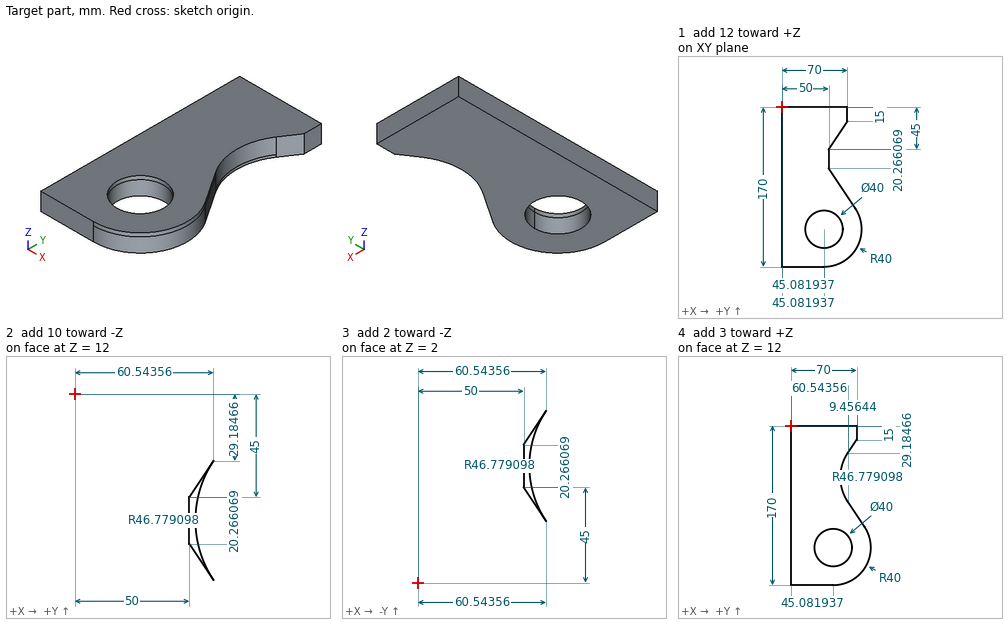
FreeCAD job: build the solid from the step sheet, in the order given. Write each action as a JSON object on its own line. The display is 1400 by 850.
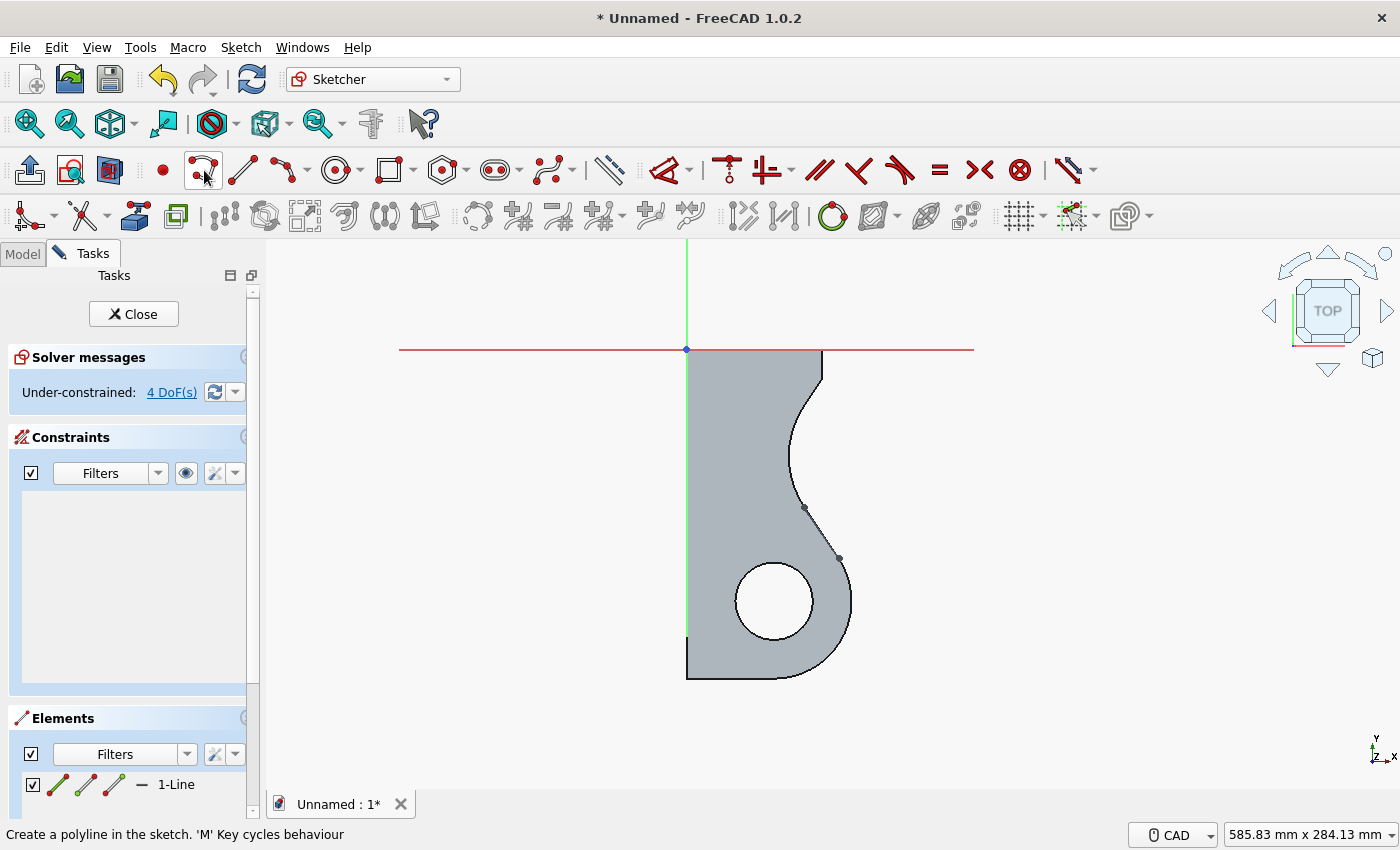
{"action": "left_click", "coordinate": [804, 406]}
{"action": "left_click", "coordinate": [822, 379]}
{"action": "left_click", "coordinate": [822, 350]}
{"action": "left_click", "coordinate": [687, 350]}
{"action": "left_click", "coordinate": [696, 679]}
{"action": "left_click", "coordinate": [774, 679]}
{"action": "right_click", "coordinate": [774, 679]}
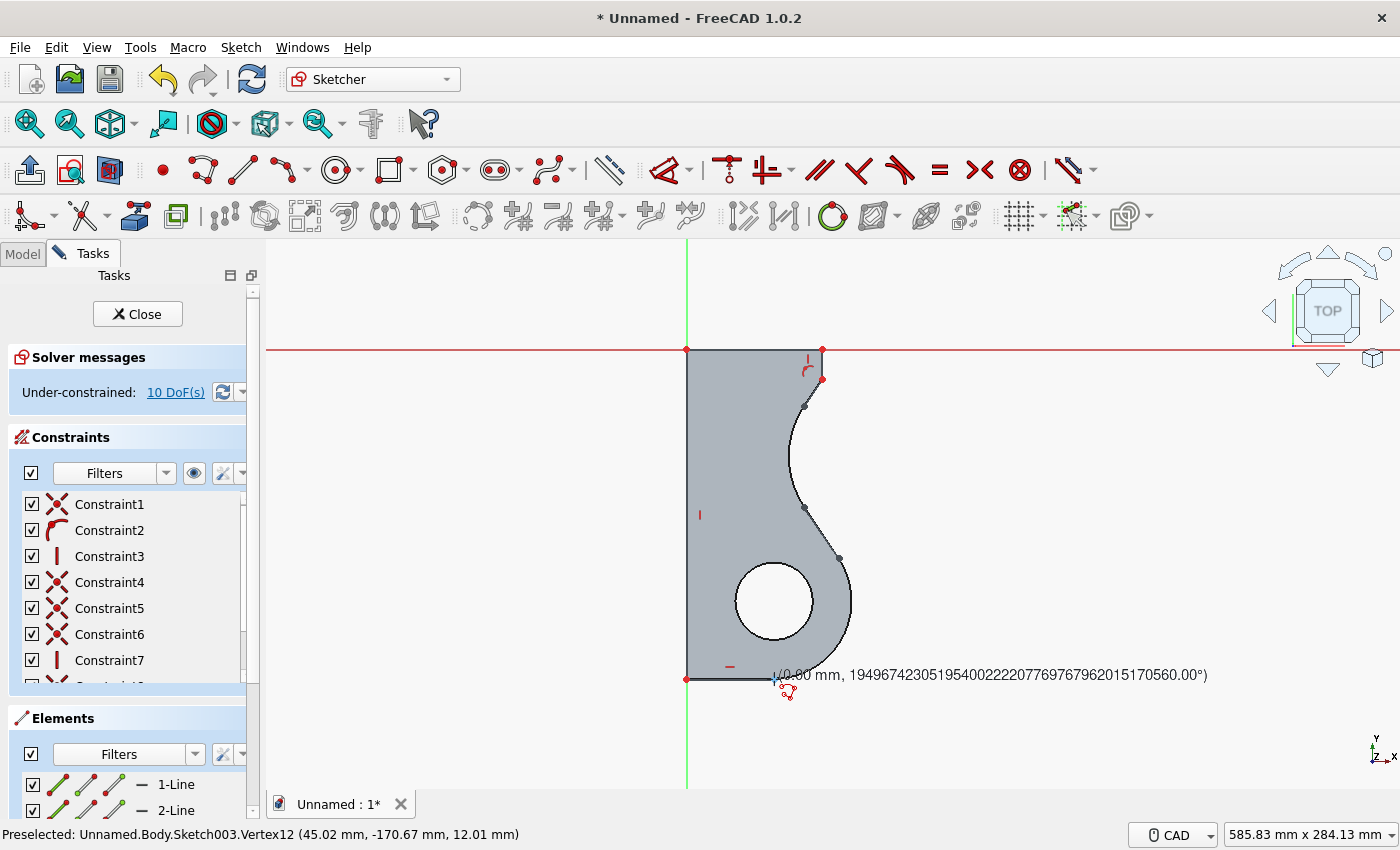
{"action": "left_click", "coordinate": [284, 170]}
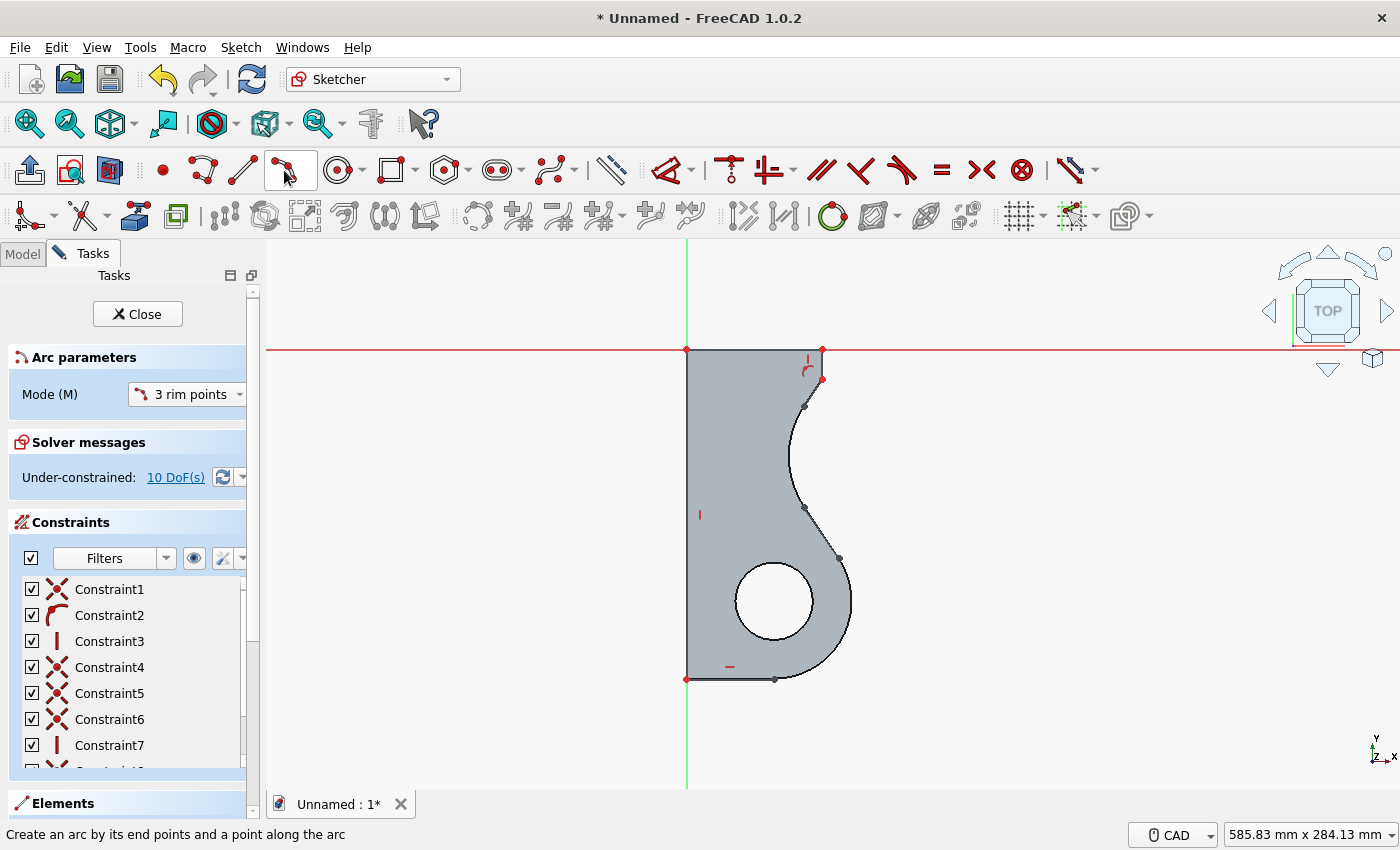
{"action": "left_click", "coordinate": [804, 508]}
{"action": "left_click", "coordinate": [804, 407]}
{"action": "left_click", "coordinate": [789, 456]}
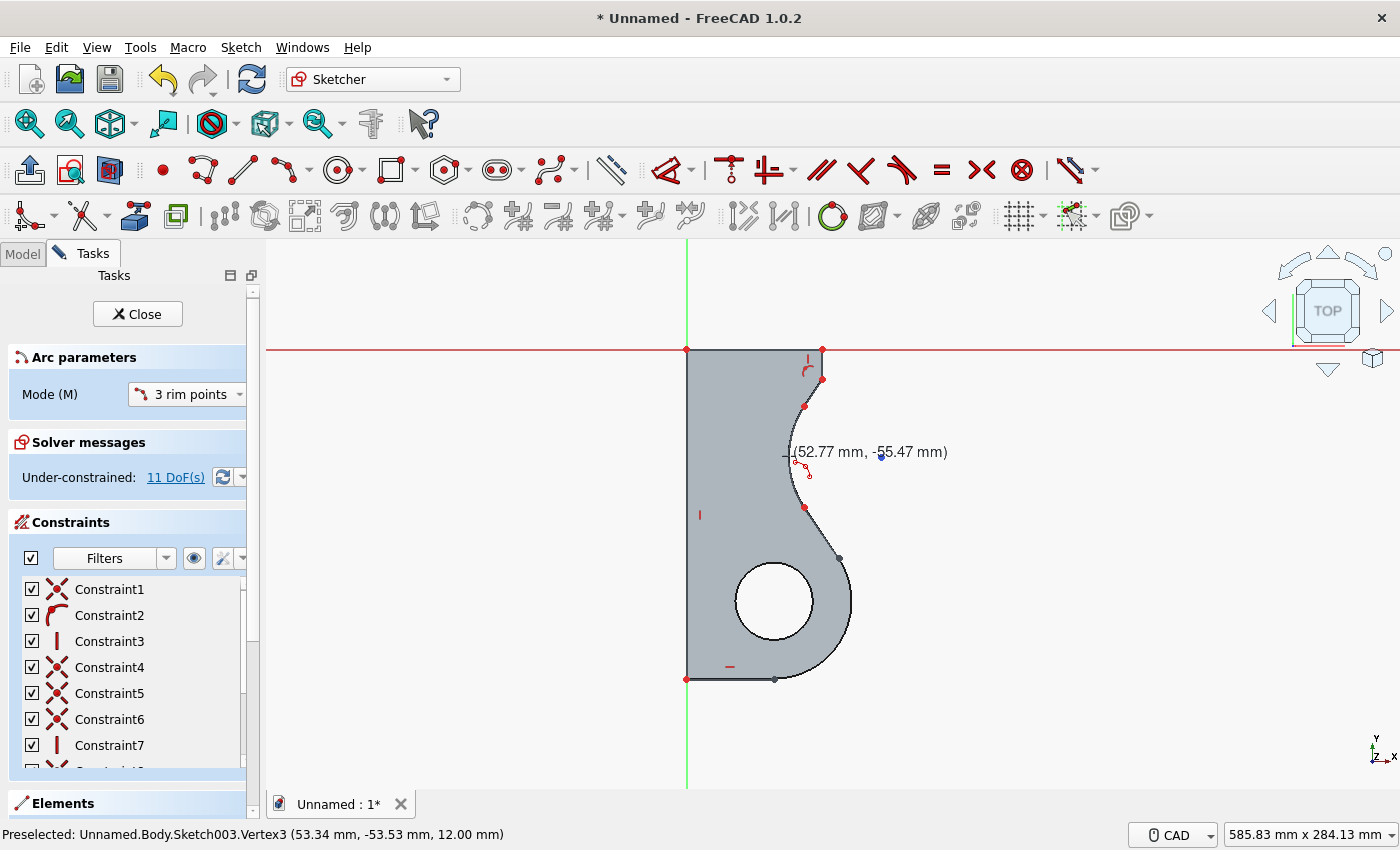
{"action": "left_click", "coordinate": [774, 680]}
{"action": "left_click", "coordinate": [839, 559]}
{"action": "left_click", "coordinate": [842, 638]}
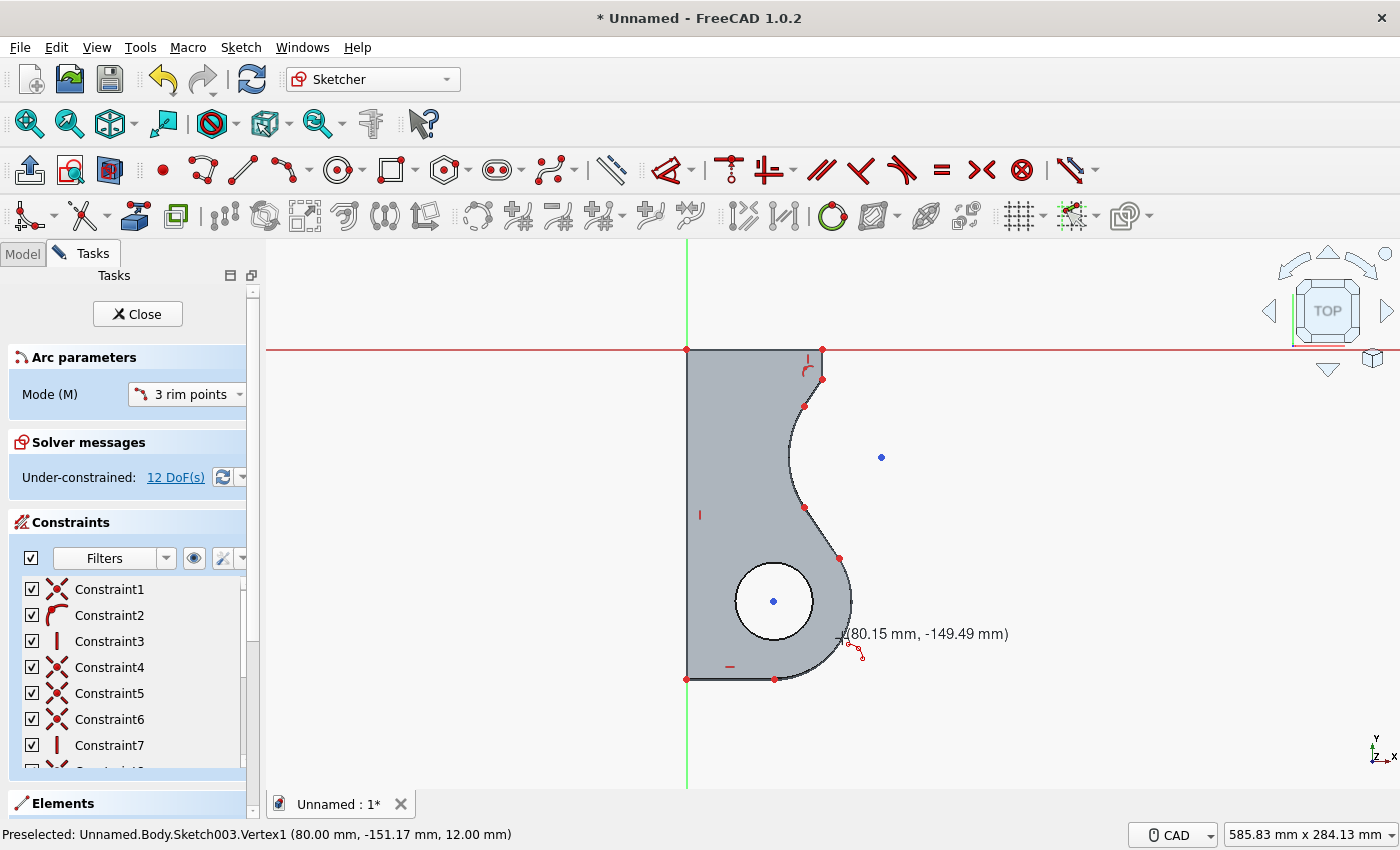
{"action": "left_click", "coordinate": [338, 170]}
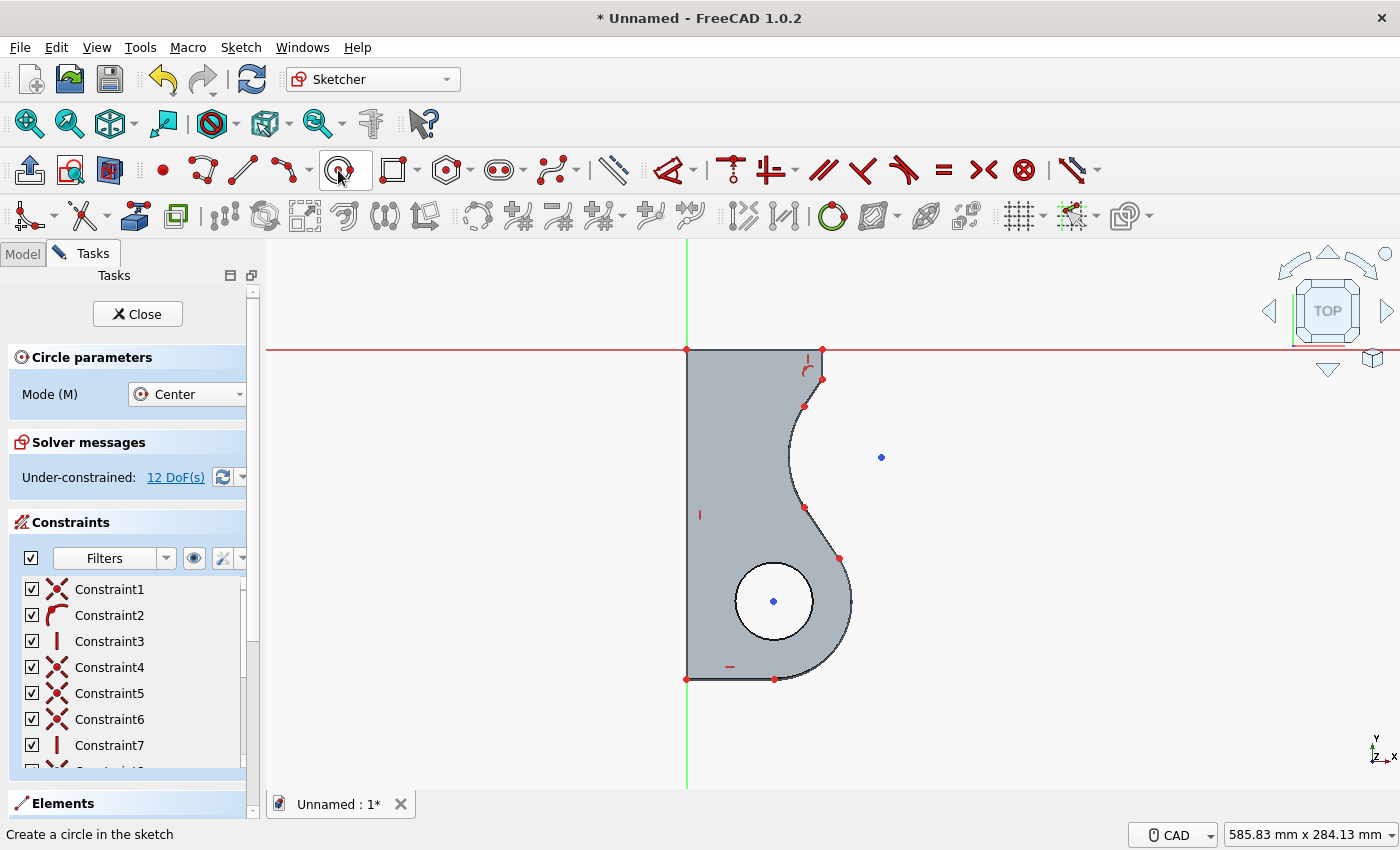
{"action": "left_click", "coordinate": [774, 601]}
{"action": "left_click", "coordinate": [801, 574]}
{"action": "key", "text": "Escape"}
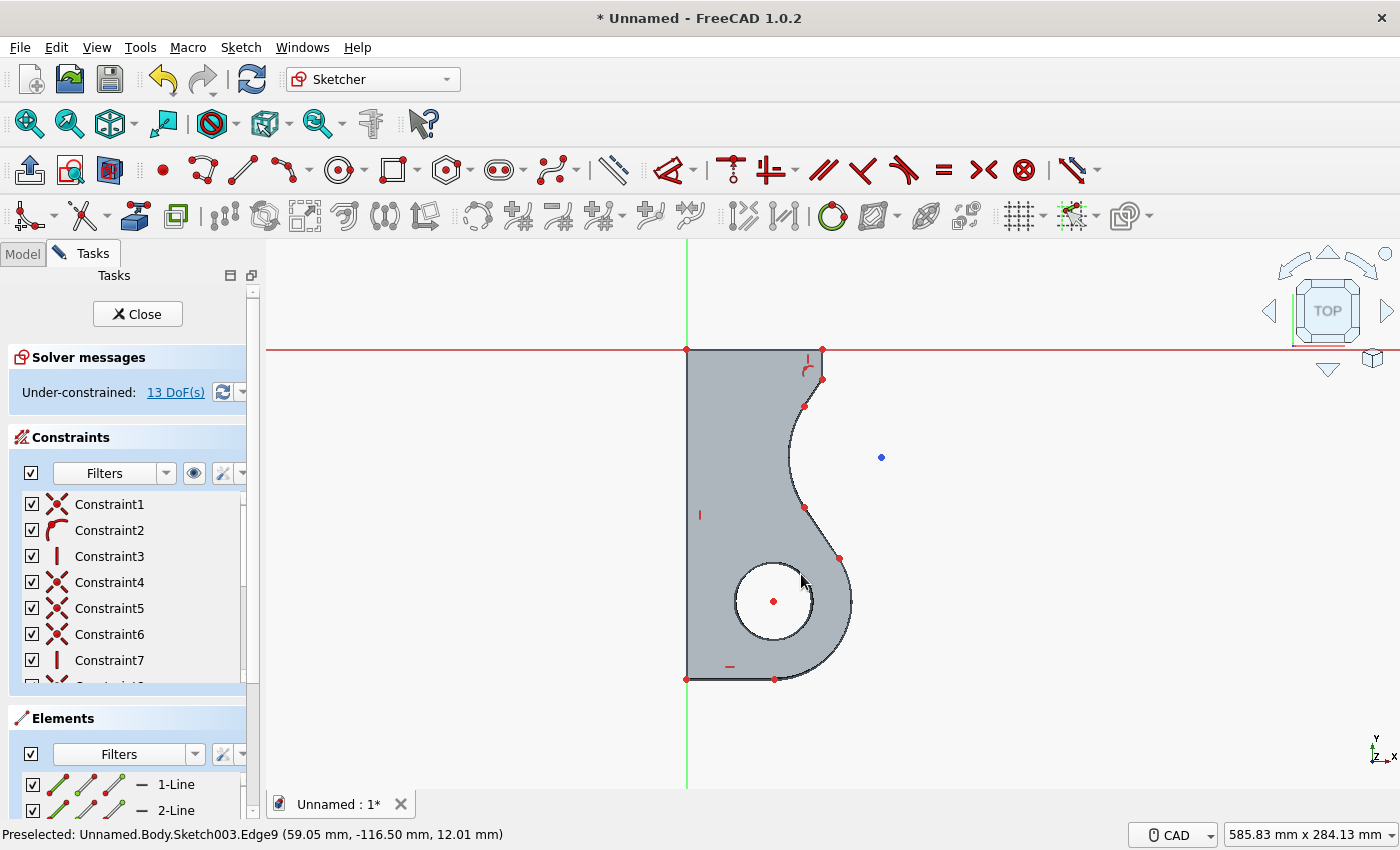
{"action": "left_click", "coordinate": [828, 544]}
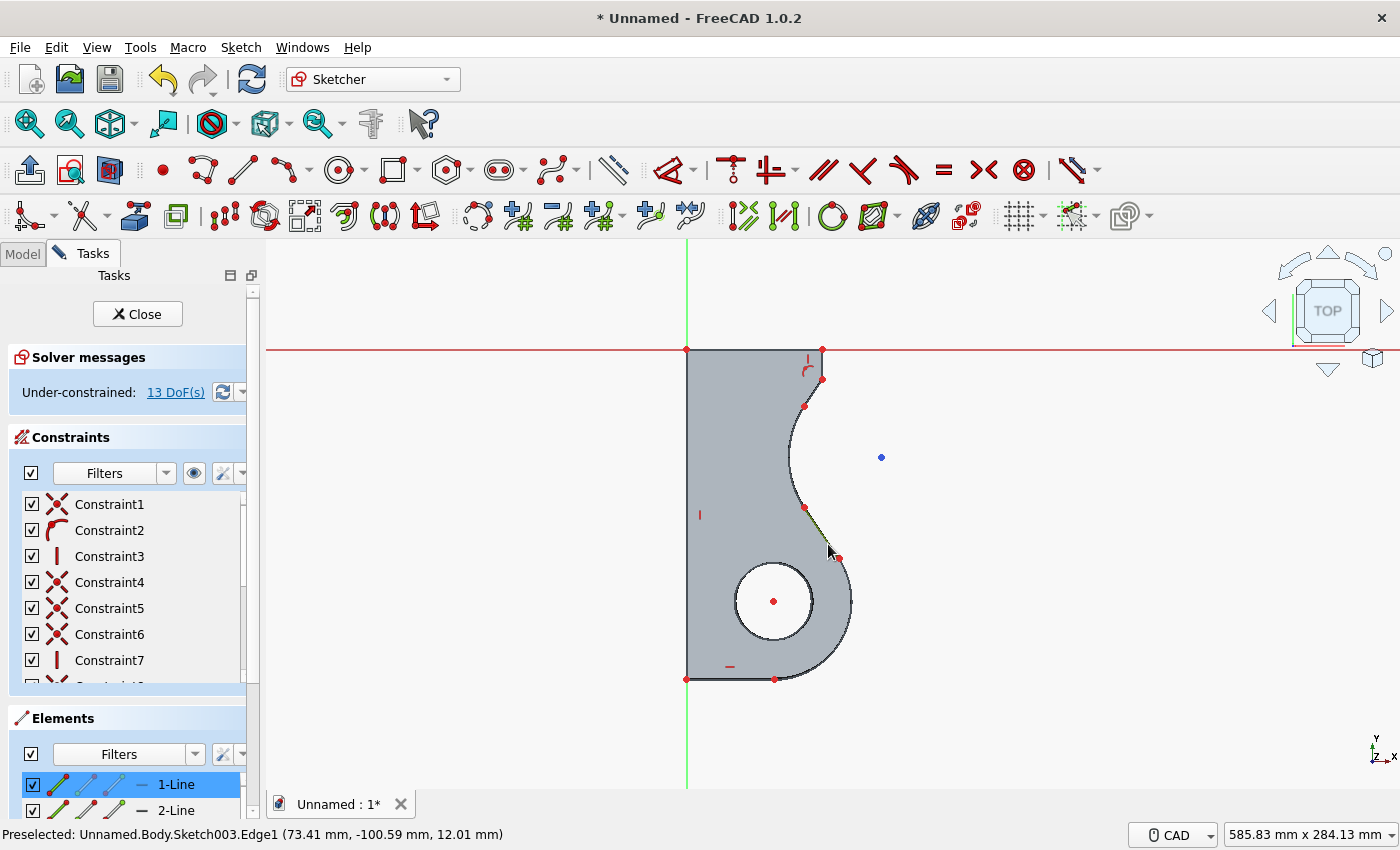
{"action": "left_click", "coordinate": [791, 436]}